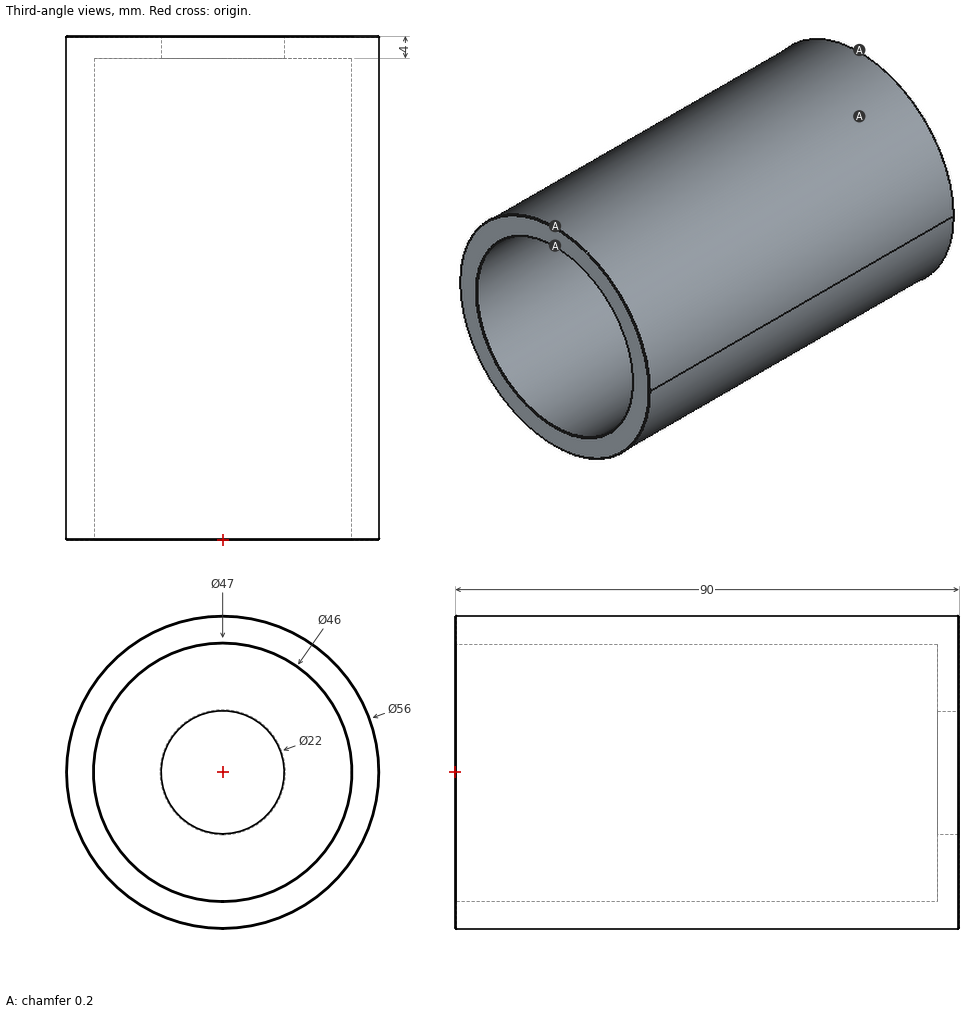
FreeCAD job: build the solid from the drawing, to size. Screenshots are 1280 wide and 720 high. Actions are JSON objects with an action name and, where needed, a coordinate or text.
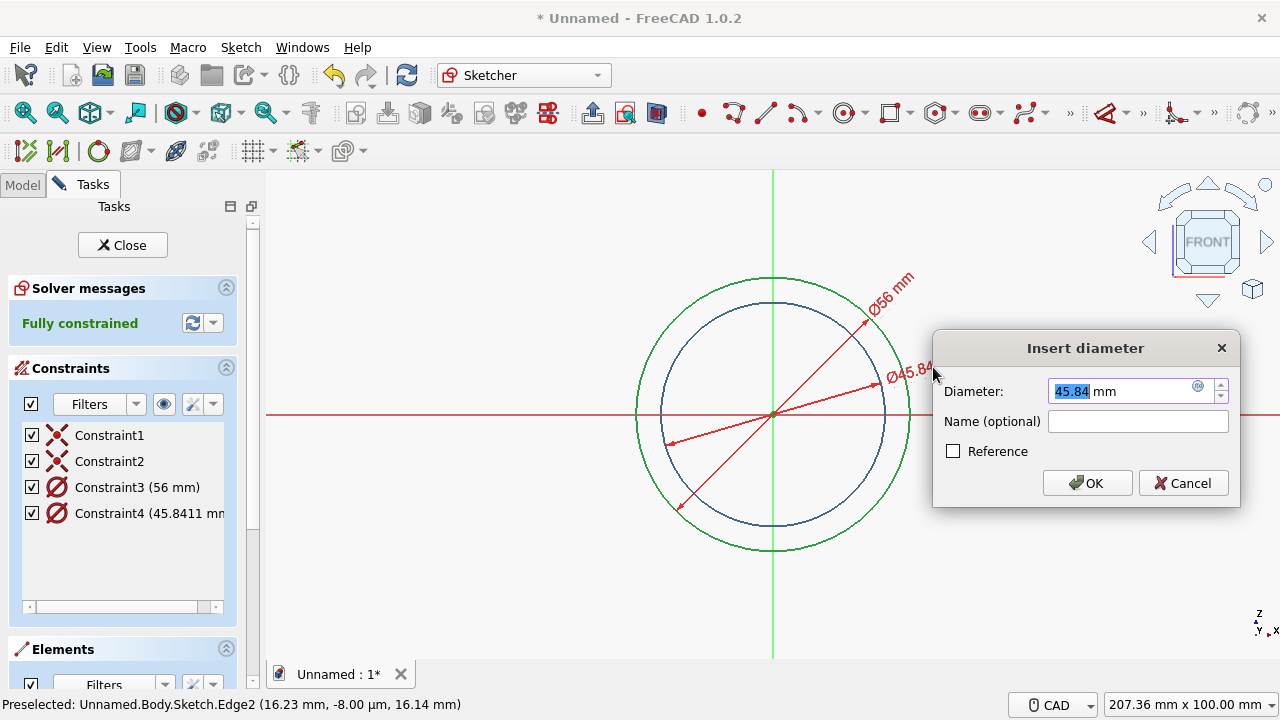
{"action": "type", "text": "46"}
{"action": "key", "text": "Return"}
{"action": "key", "text": "Escape"}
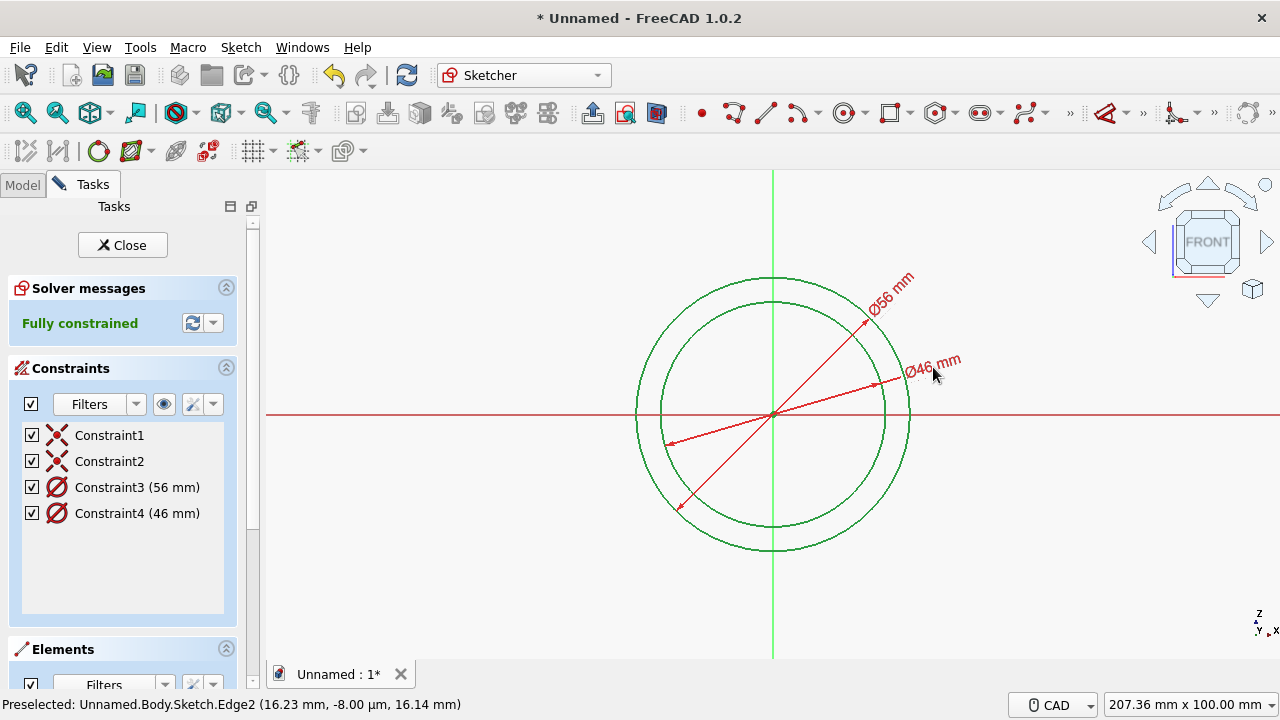
{"action": "left_click", "coordinate": [123, 245]}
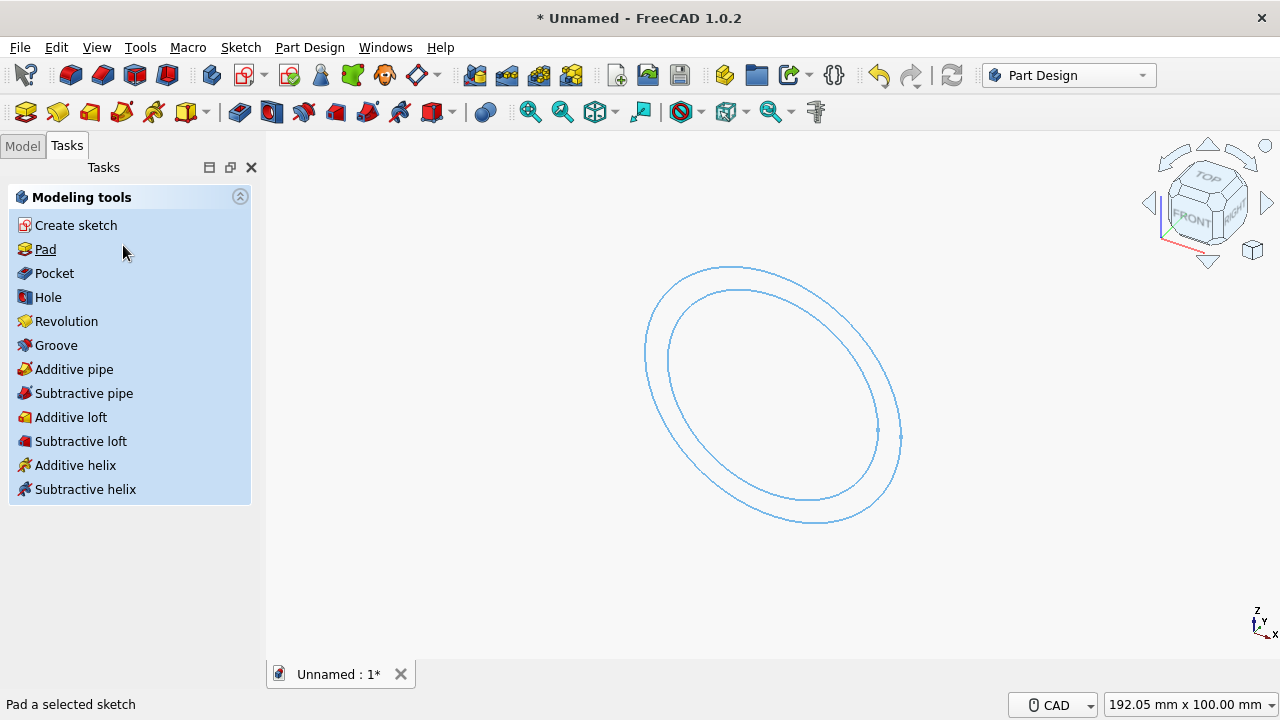
{"action": "left_click", "coordinate": [26, 112]}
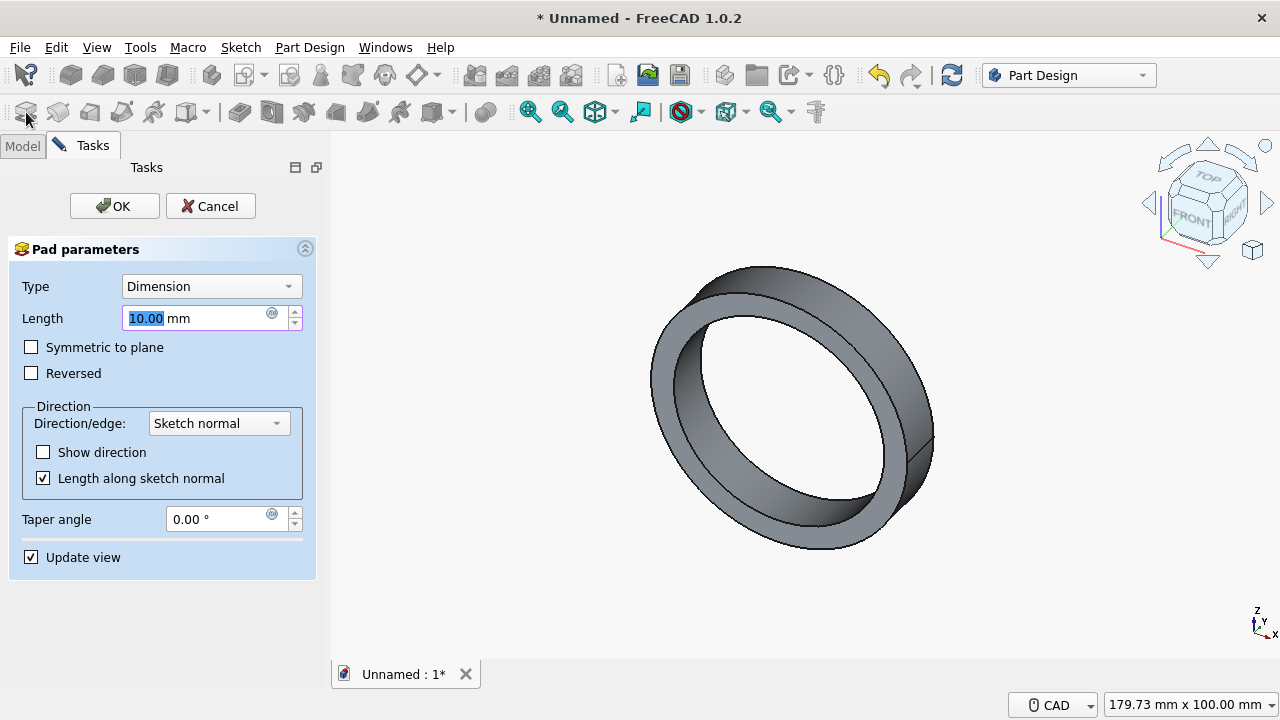
{"action": "type", "text": "90"}
{"action": "key", "text": "Tab"}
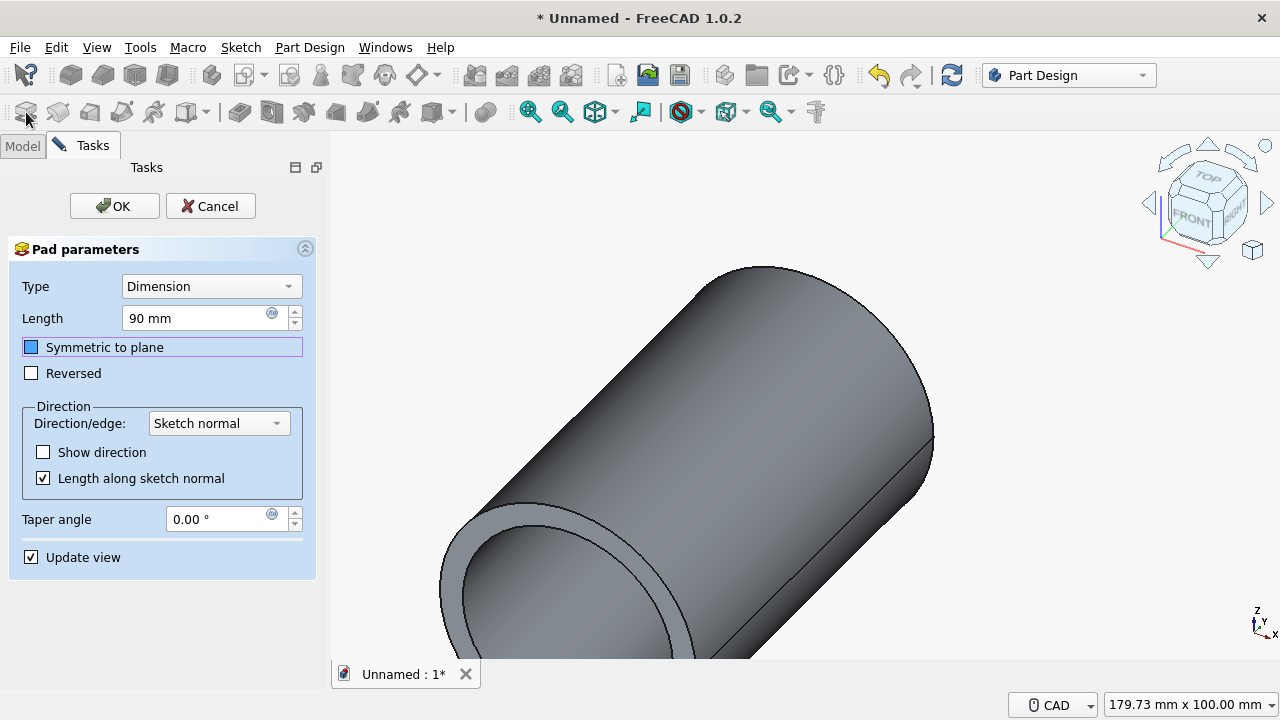
{"action": "left_click", "coordinate": [30, 373]}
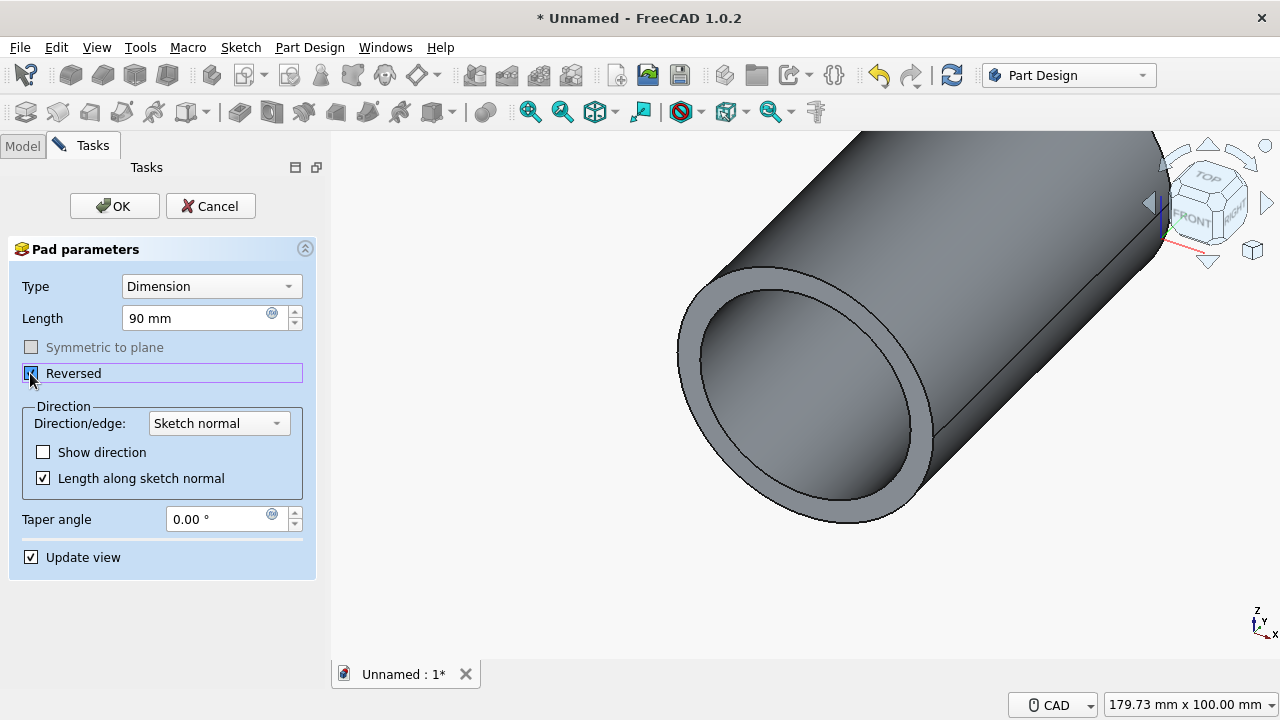
{"action": "left_click", "coordinate": [115, 206]}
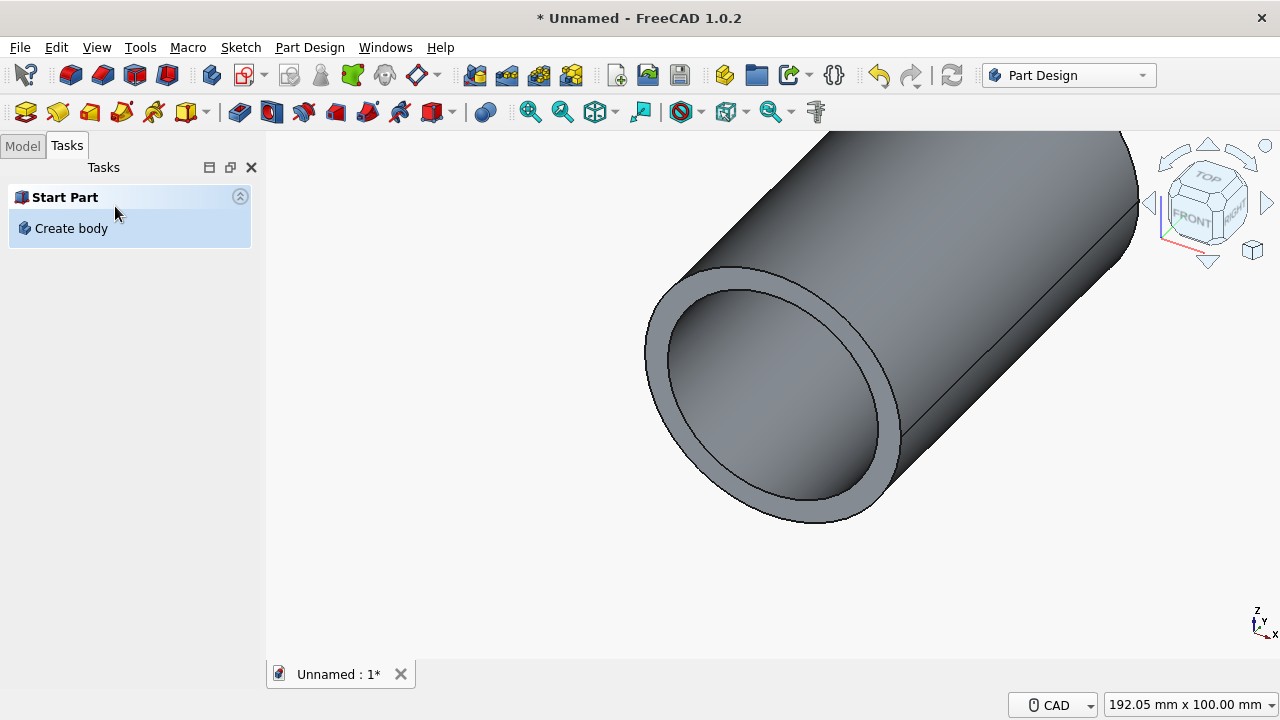
{"action": "key", "text": "v f"}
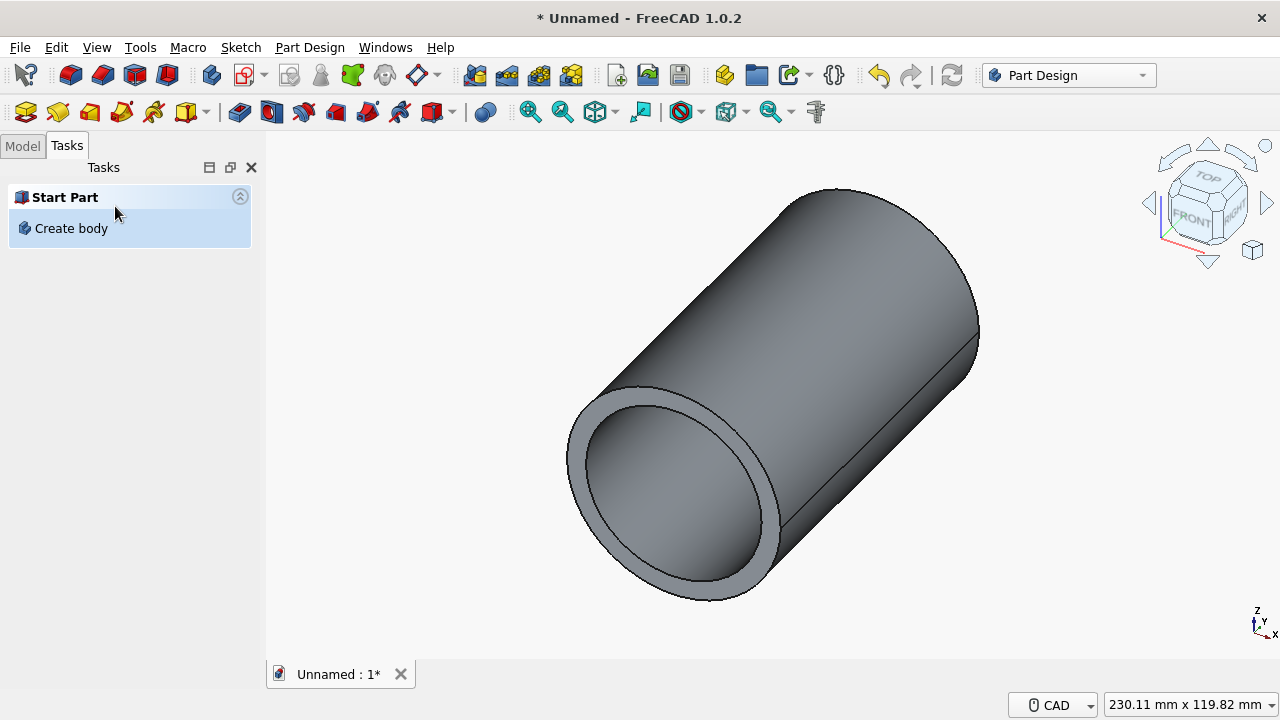
{"action": "key", "text": "4"}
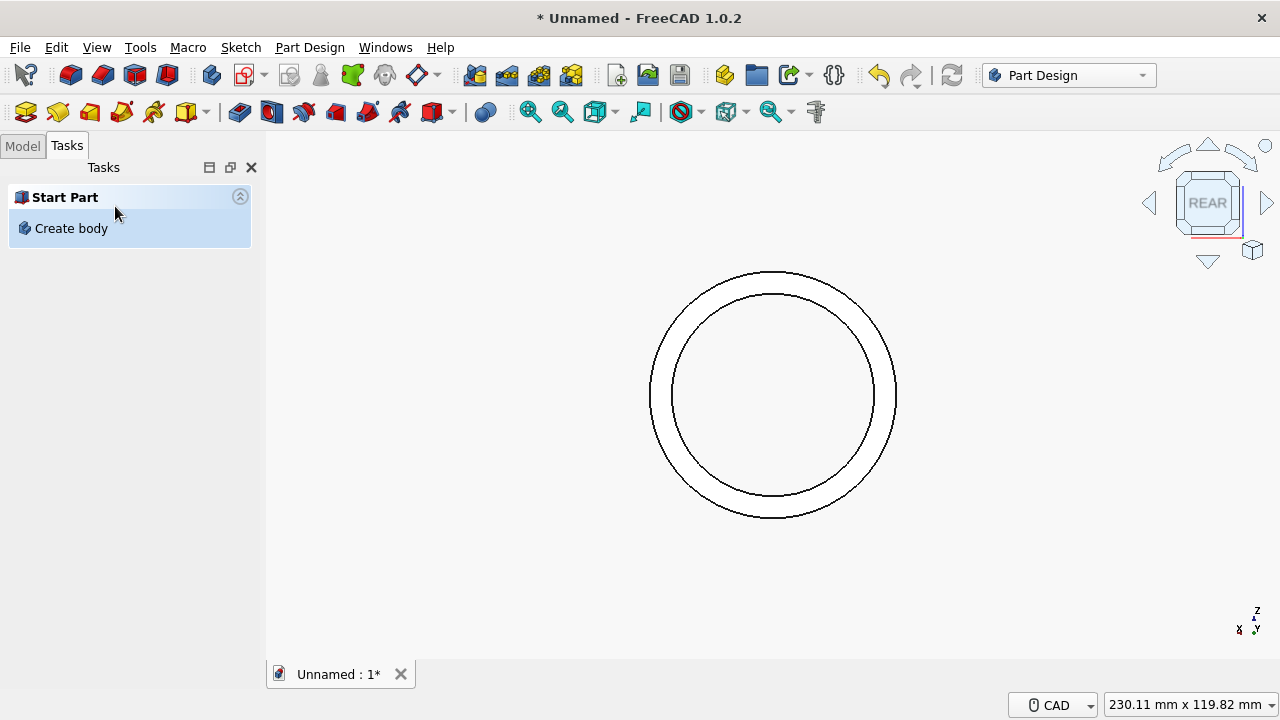
{"action": "left_click", "coordinate": [879, 429]}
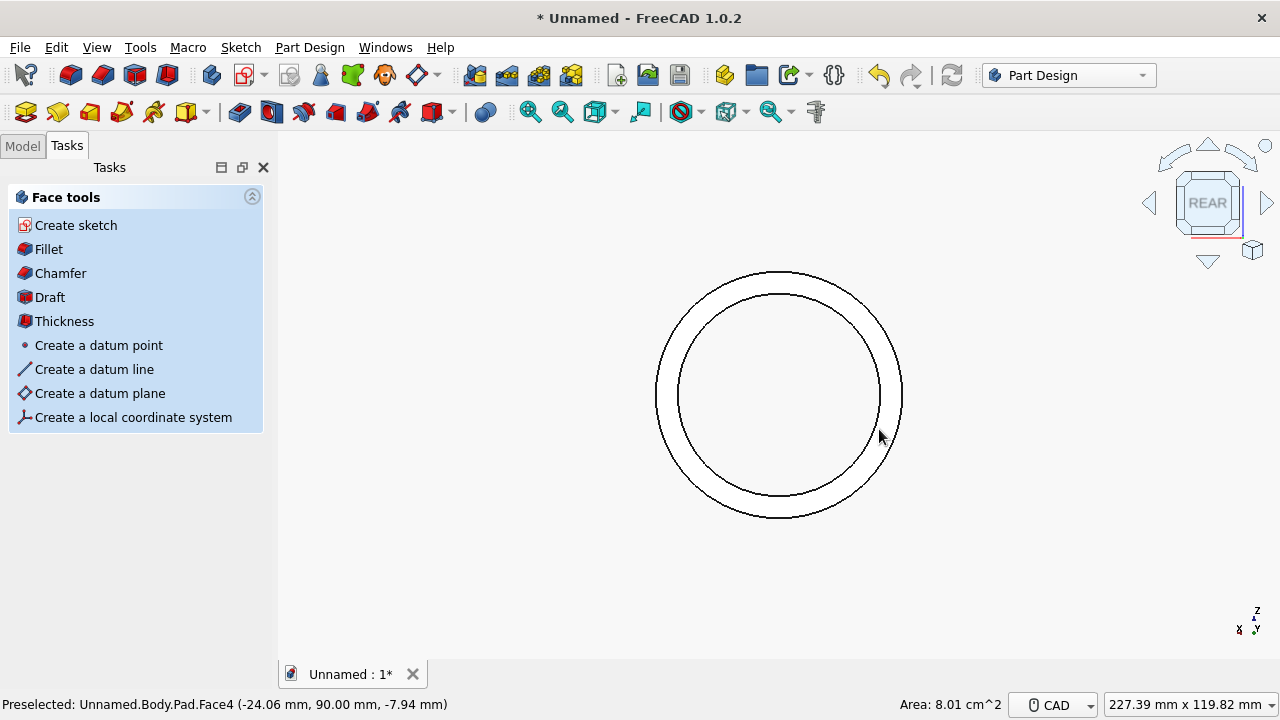
{"action": "left_click", "coordinate": [244, 76]}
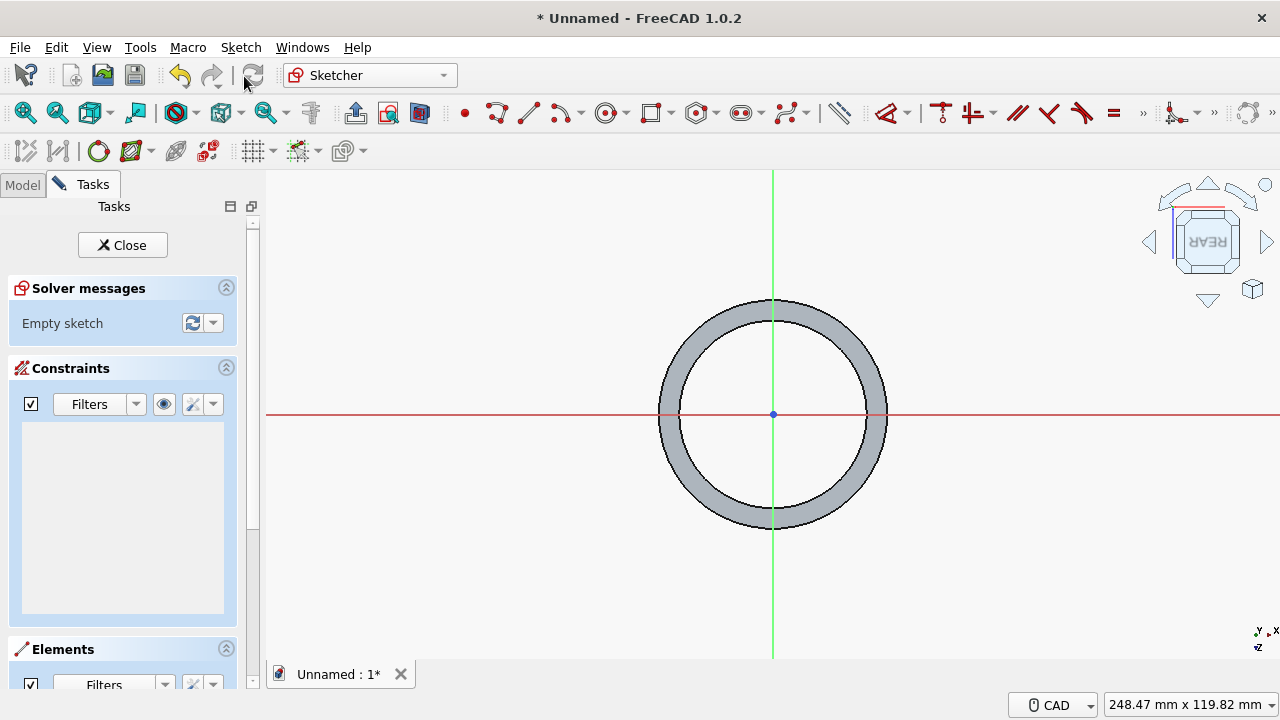
{"action": "scroll", "coordinate": [912, 414], "scroll_direction": "up", "scroll_amount": 2}